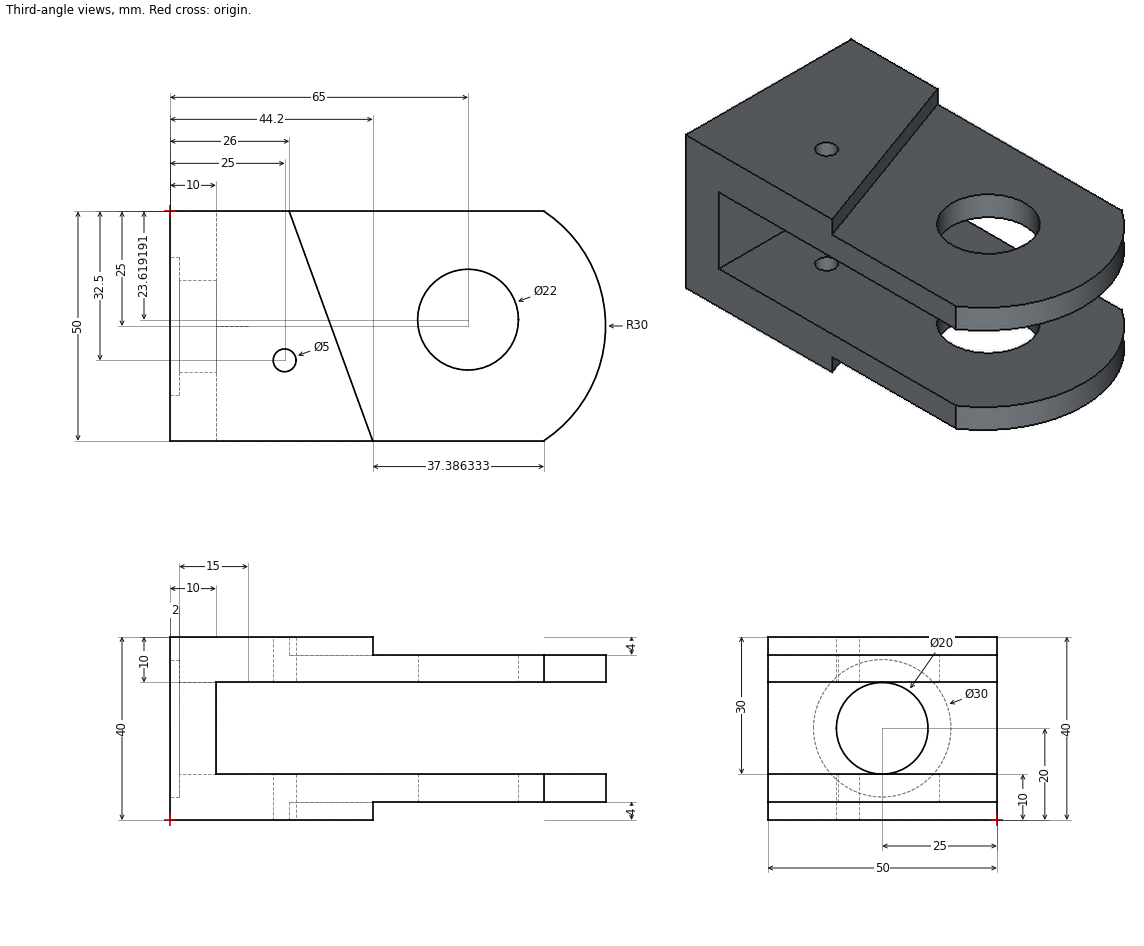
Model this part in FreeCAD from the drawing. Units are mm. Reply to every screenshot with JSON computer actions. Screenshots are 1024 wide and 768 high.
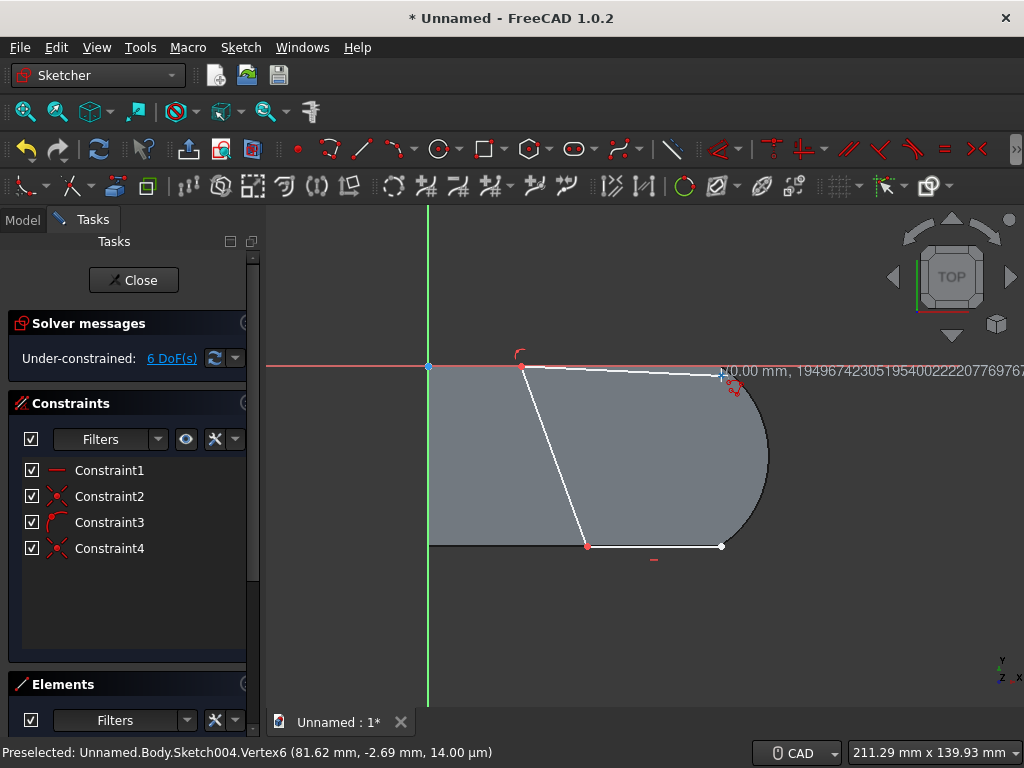
{"action": "key", "text": "g 3 a"}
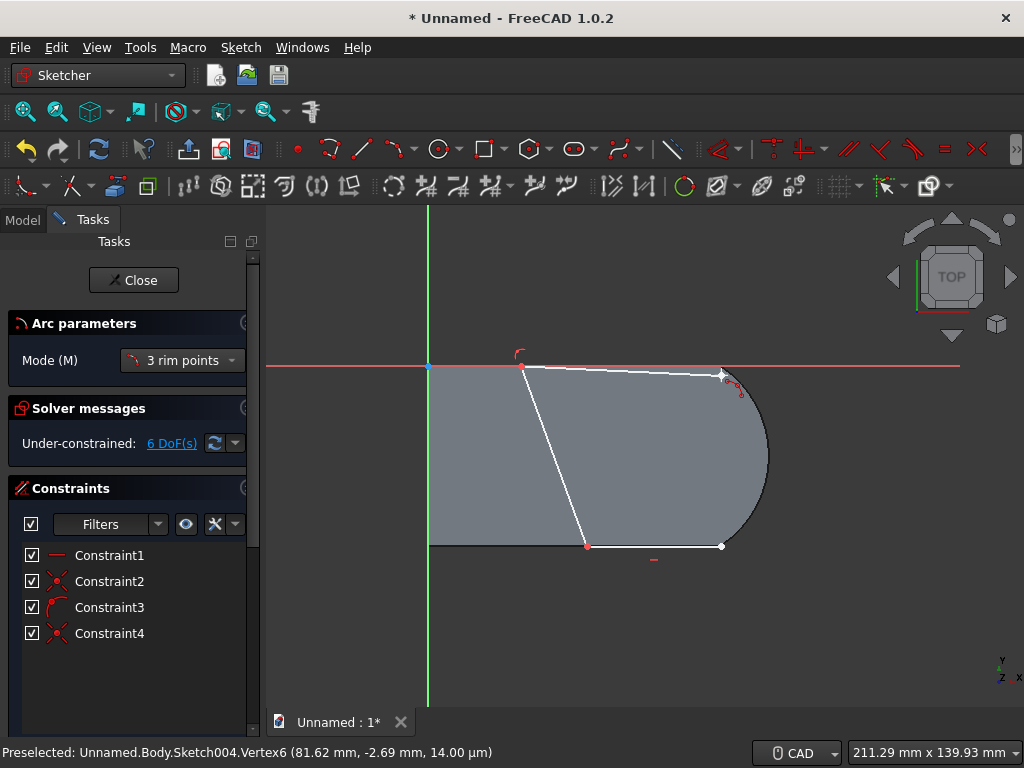
{"action": "left_click", "coordinate": [721, 376]}
{"action": "left_click", "coordinate": [721, 547]}
{"action": "left_click", "coordinate": [769, 456]}
{"action": "key", "text": "Escape"}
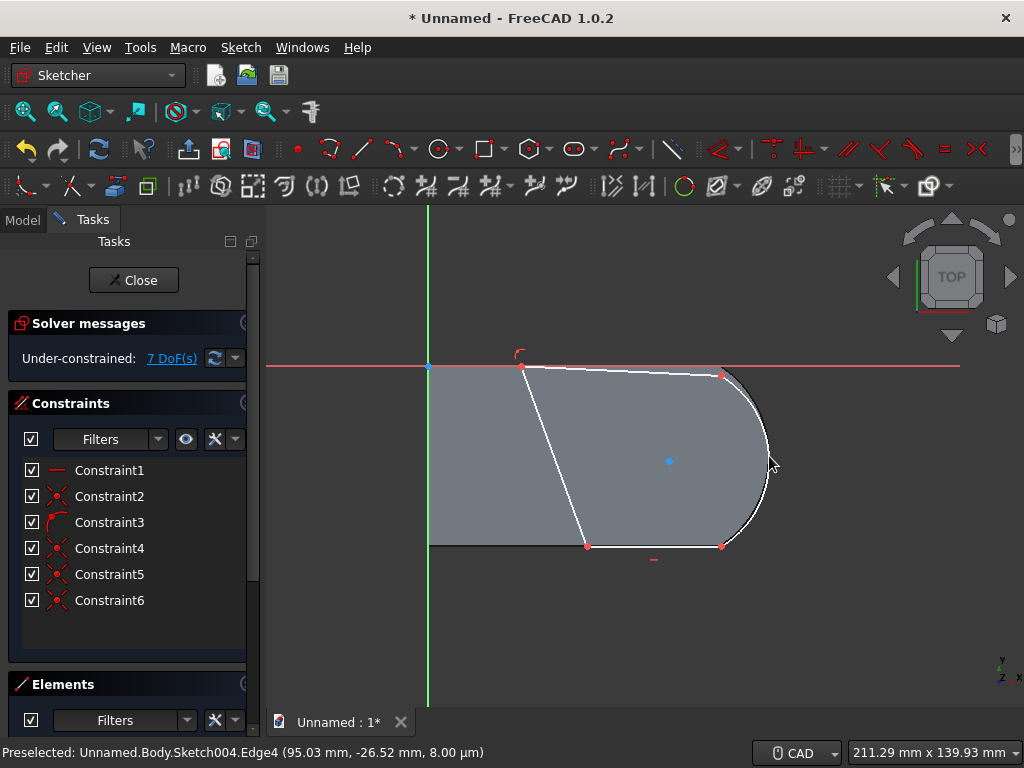
{"action": "left_click", "coordinate": [581, 369]}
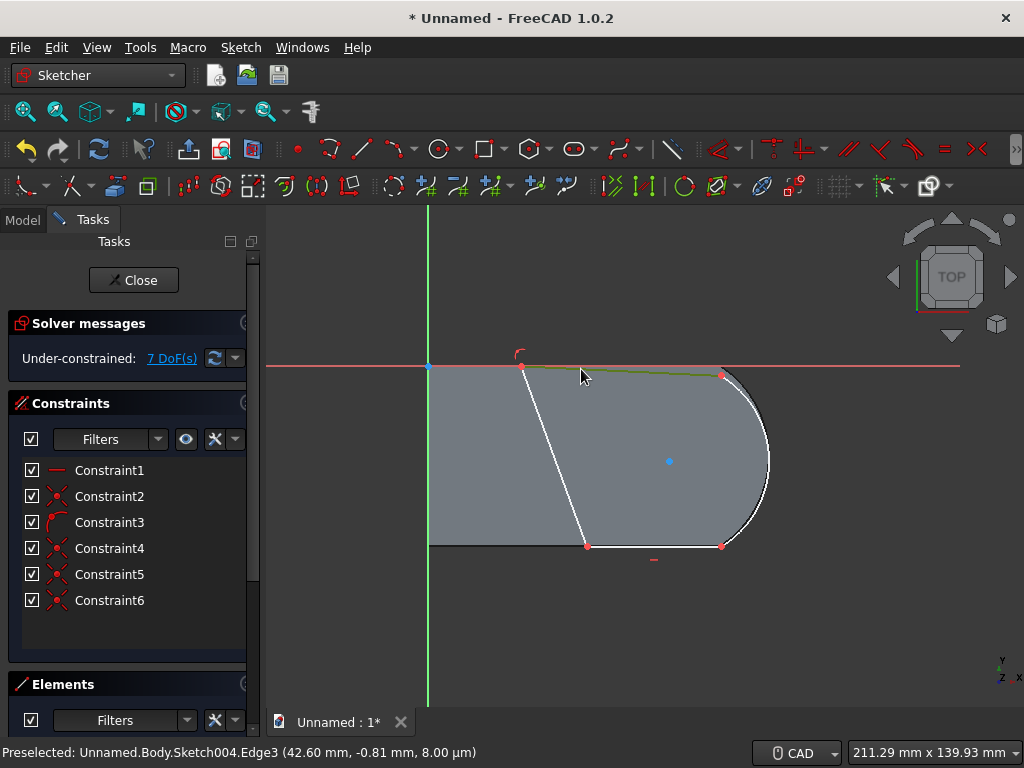
{"action": "left_click", "coordinate": [826, 150]}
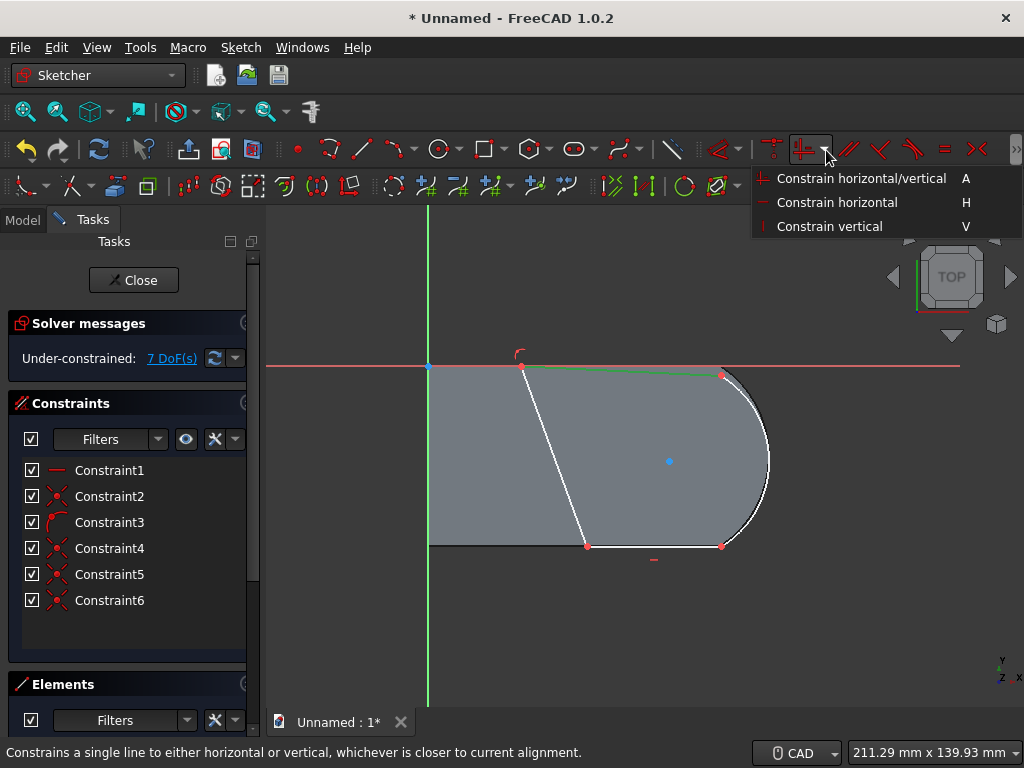
{"action": "left_click", "coordinate": [887, 202]}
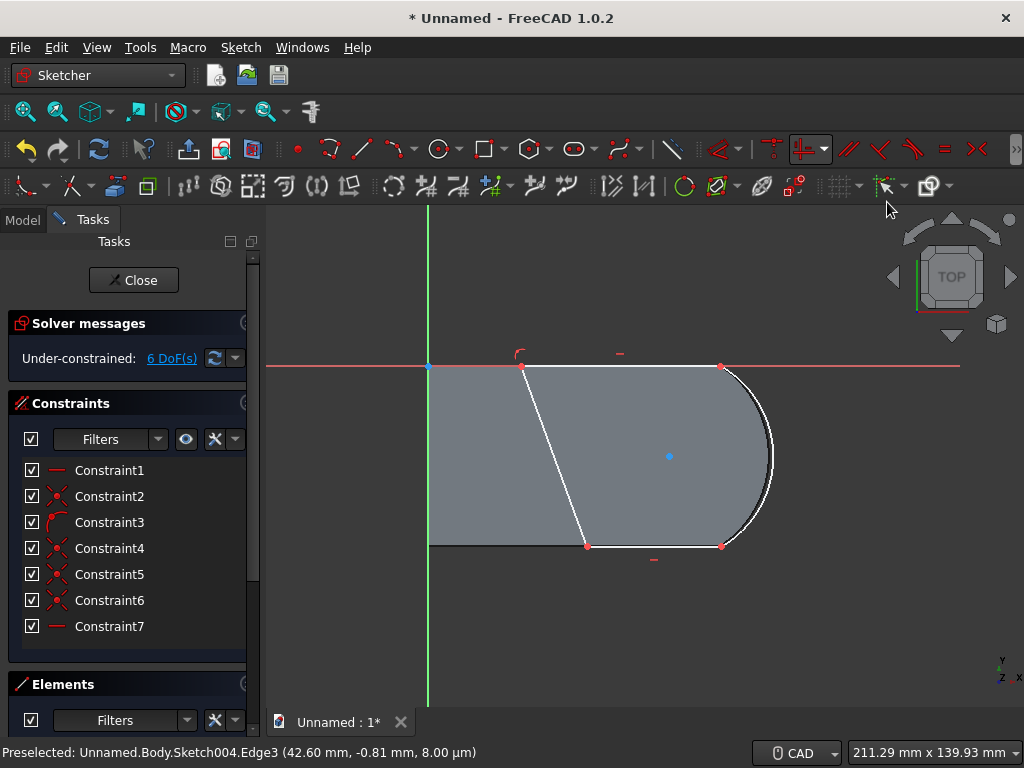
{"action": "left_click", "coordinate": [764, 499]}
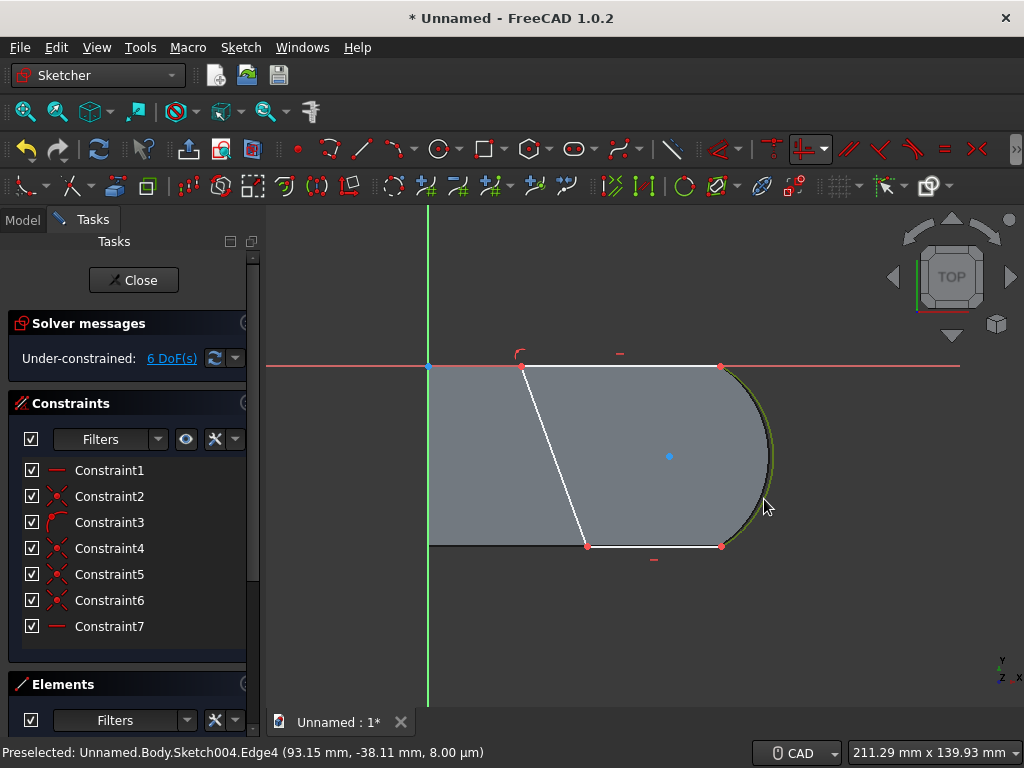
{"action": "key", "text": "k r"}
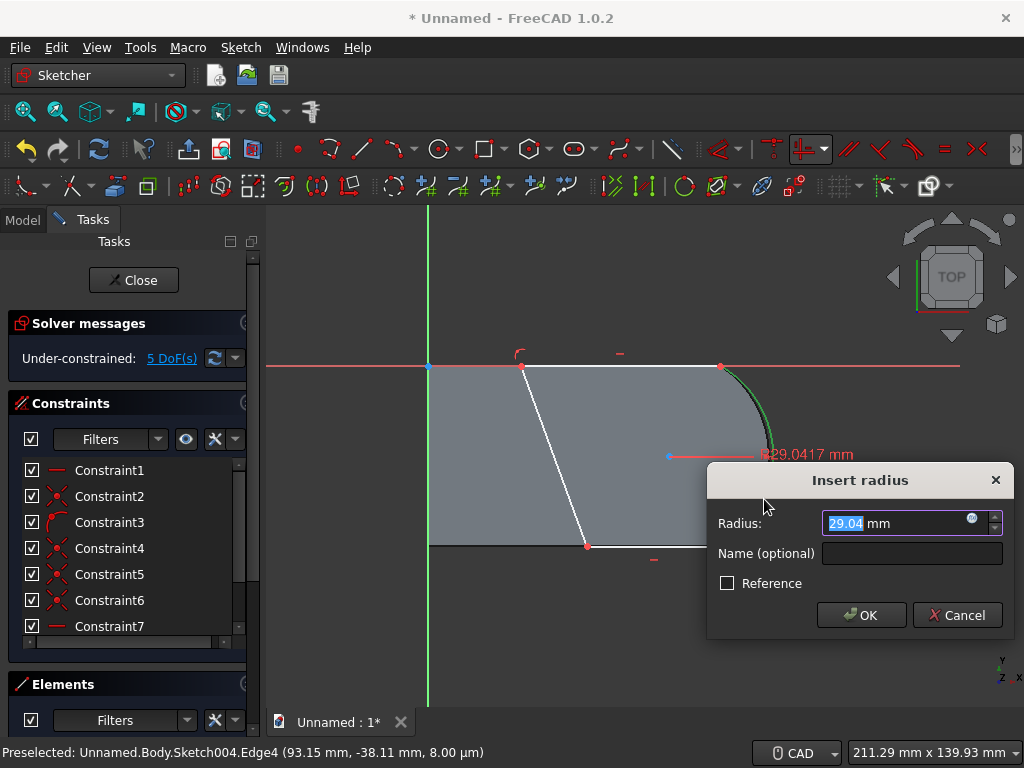
{"action": "type", "text": "30"}
{"action": "key", "text": "Return"}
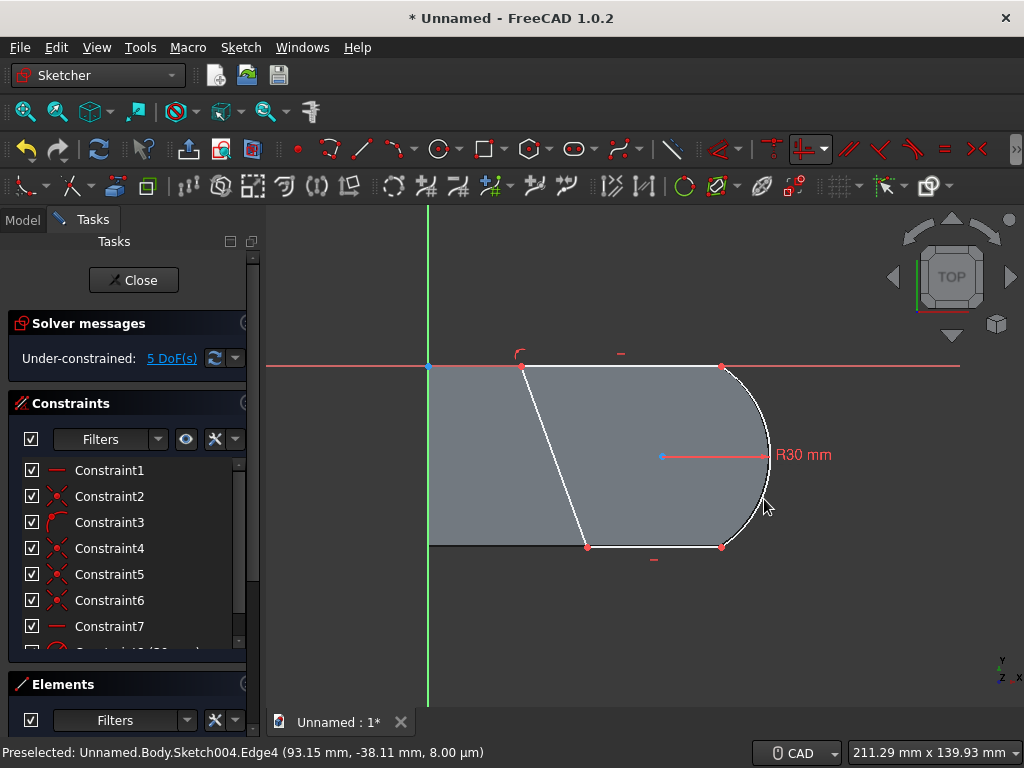
{"action": "left_click", "coordinate": [721, 547]}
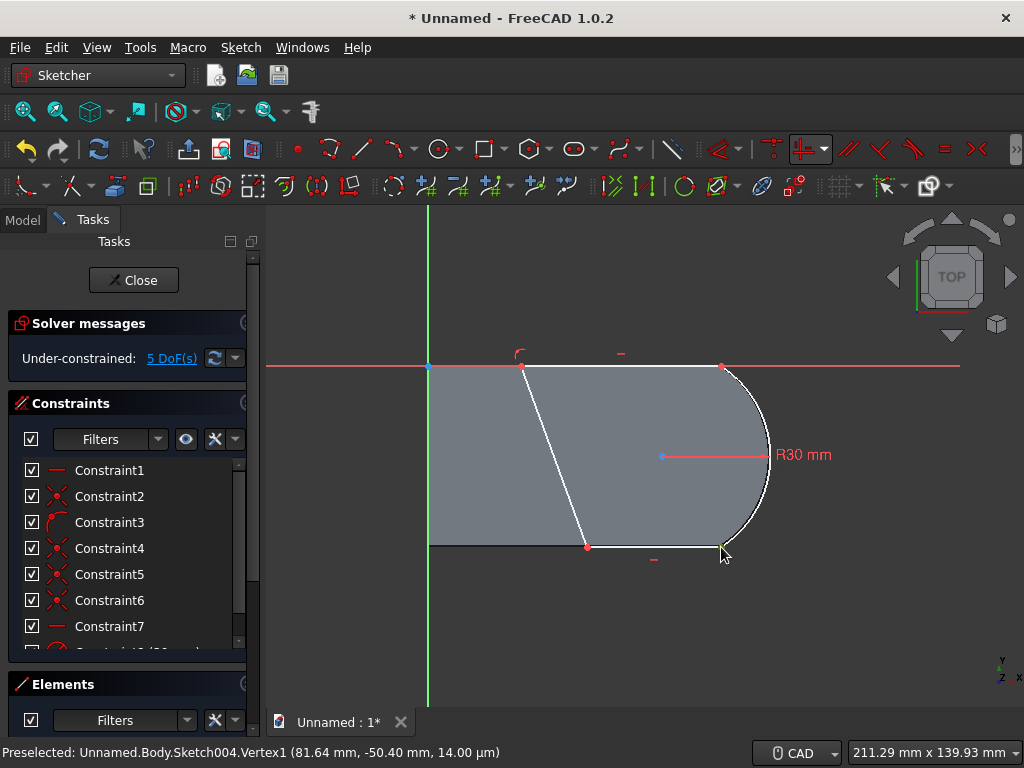
{"action": "left_click", "coordinate": [740, 150]}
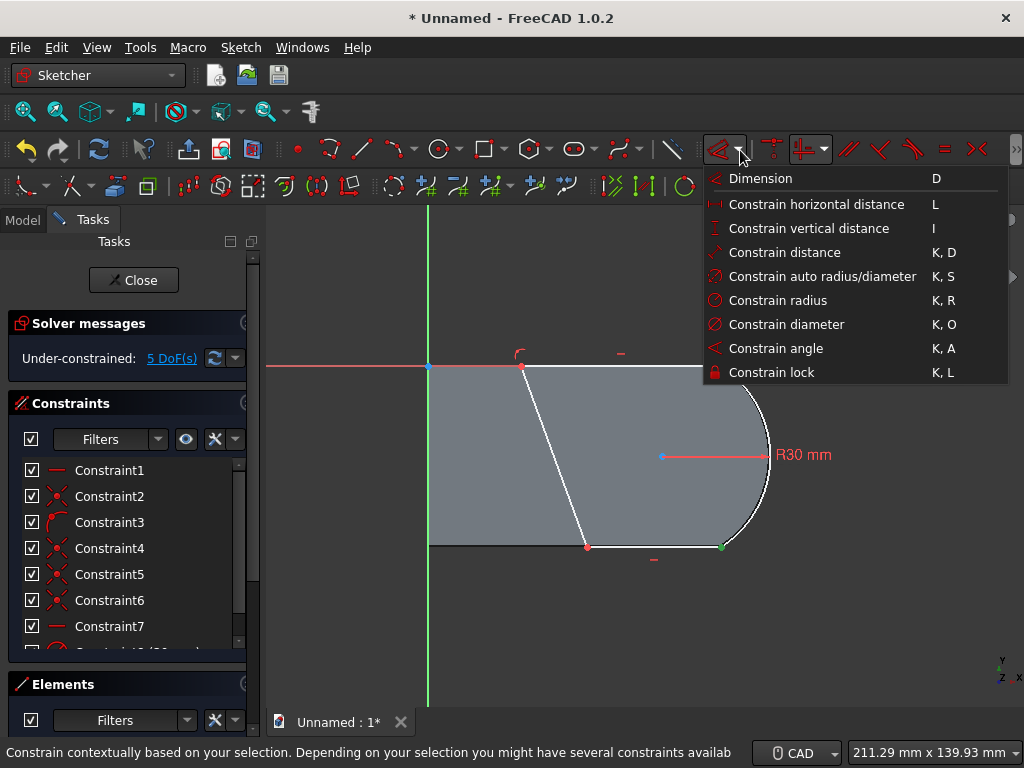
{"action": "left_click", "coordinate": [856, 228]}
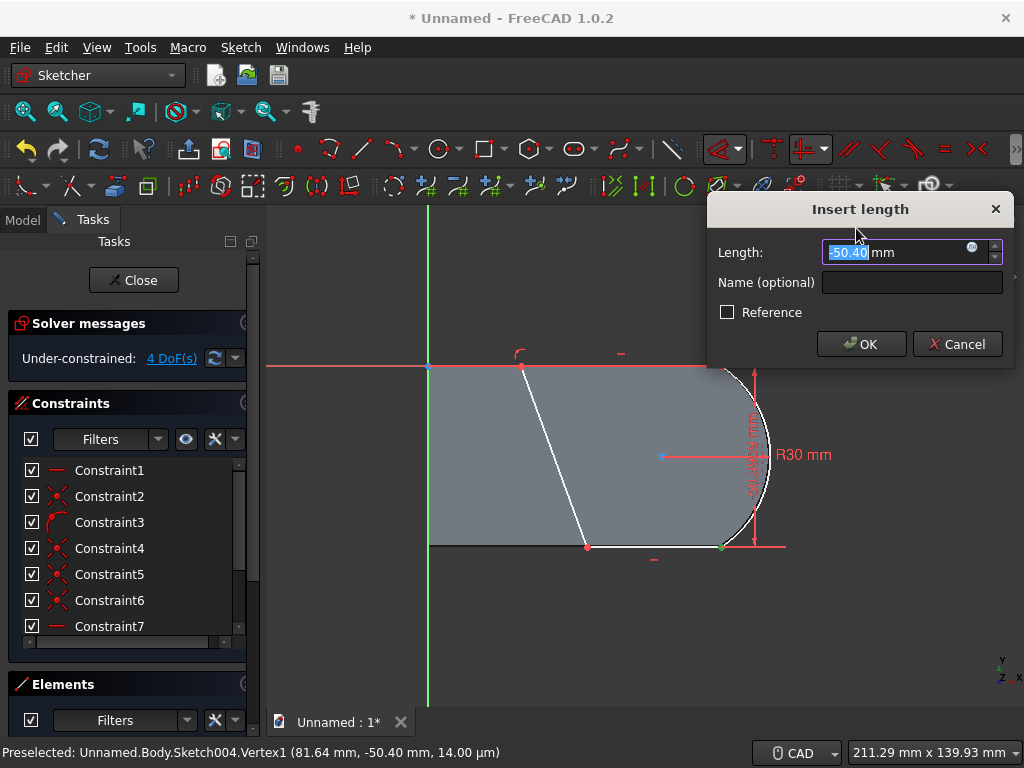
{"action": "type", "text": "-50"}
{"action": "key", "text": "Return"}